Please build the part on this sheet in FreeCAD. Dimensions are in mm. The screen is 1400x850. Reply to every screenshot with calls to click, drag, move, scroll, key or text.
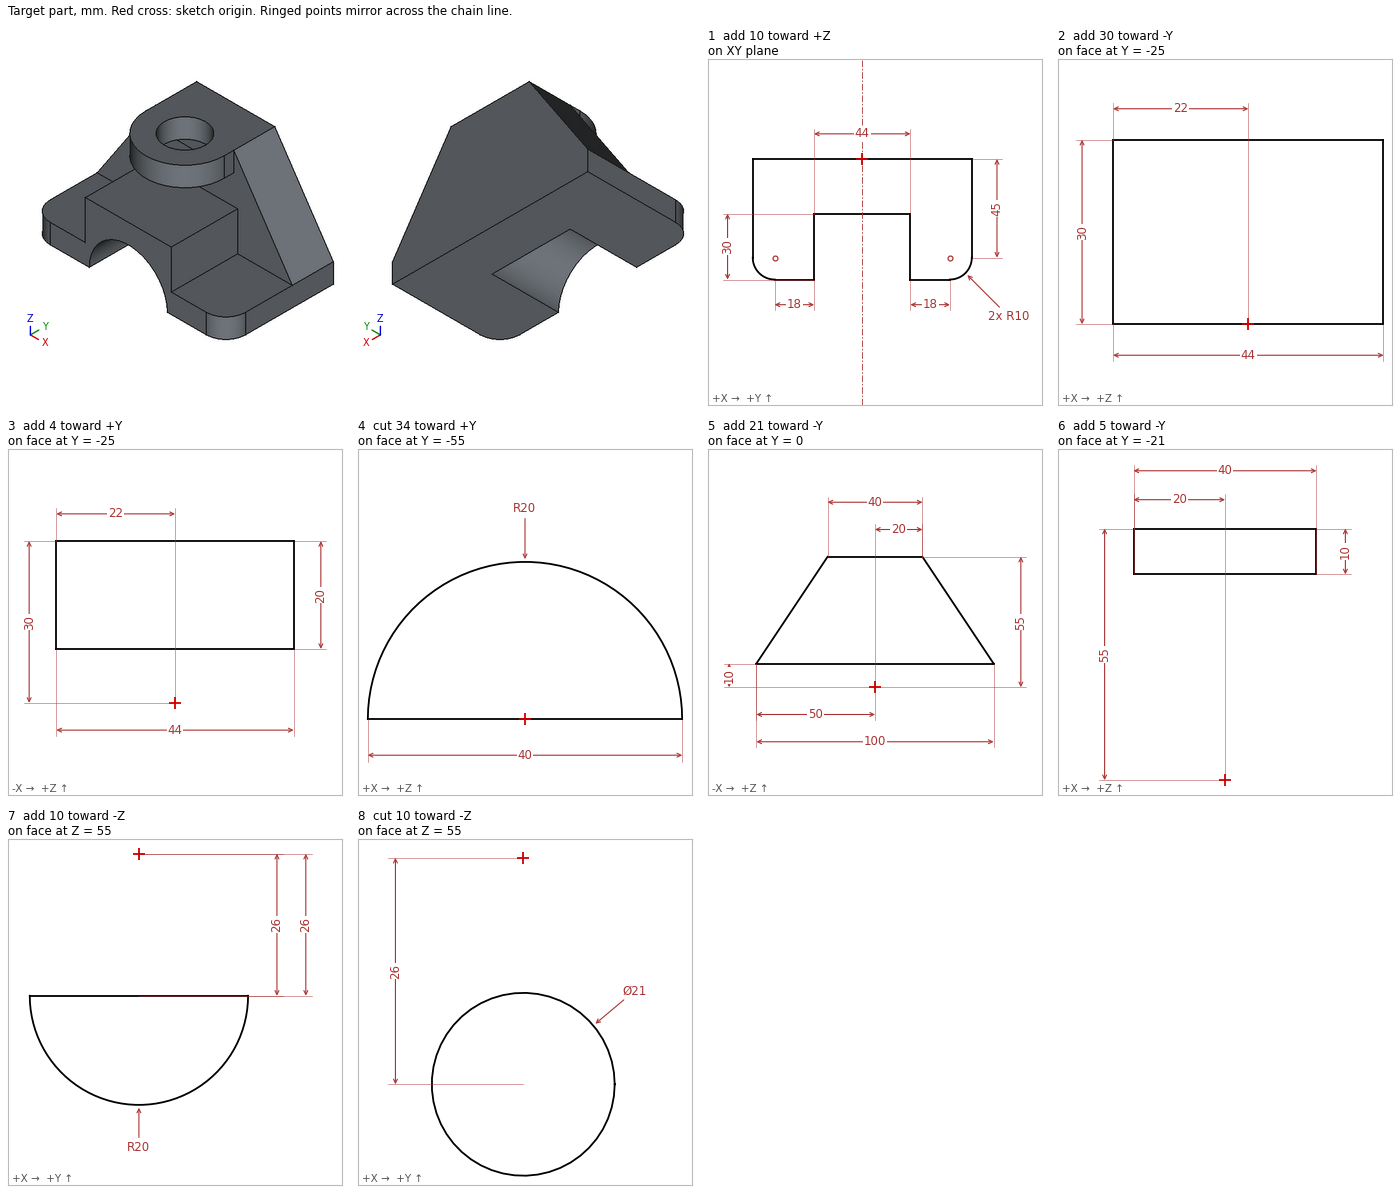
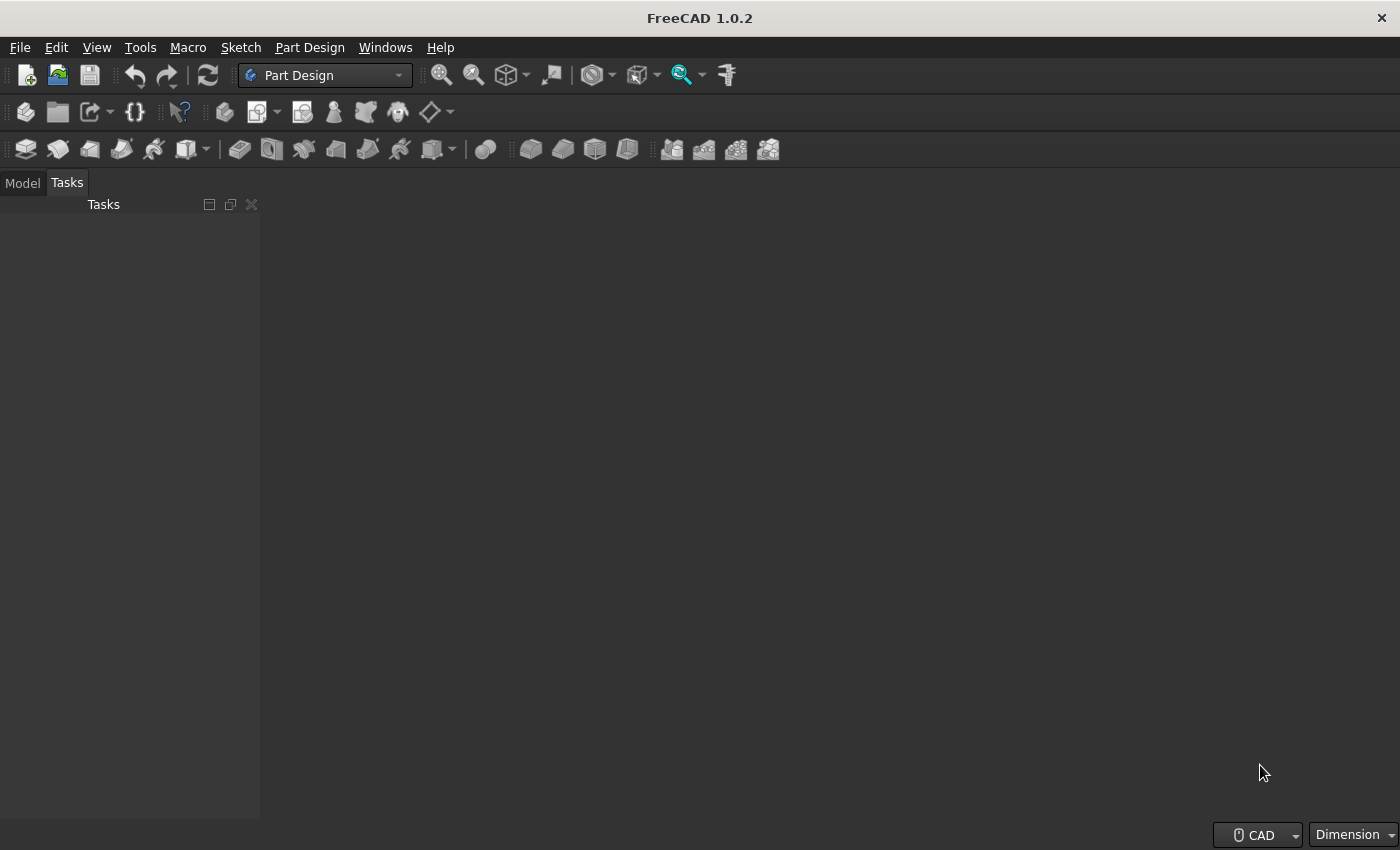
click(26, 76)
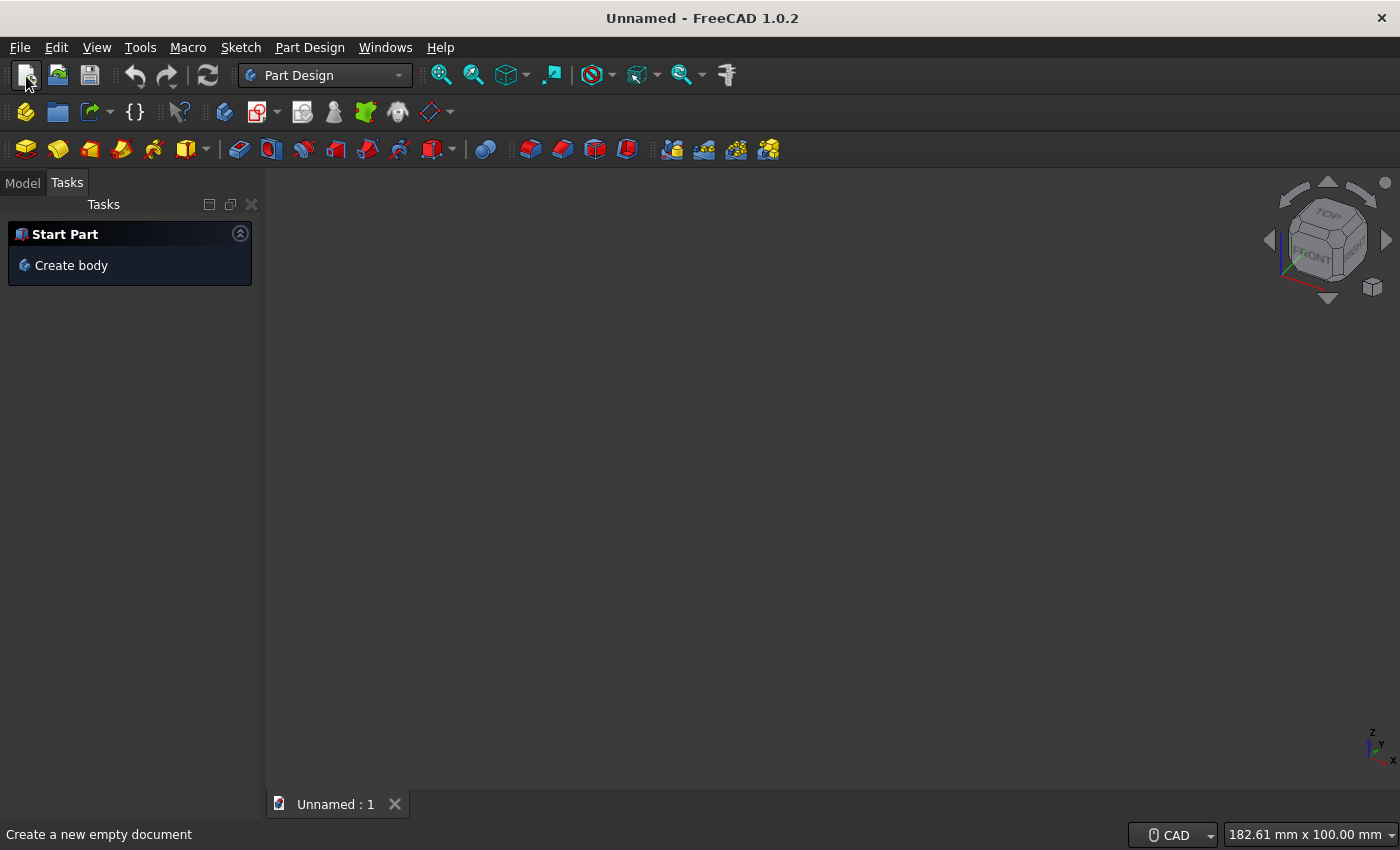
click(258, 112)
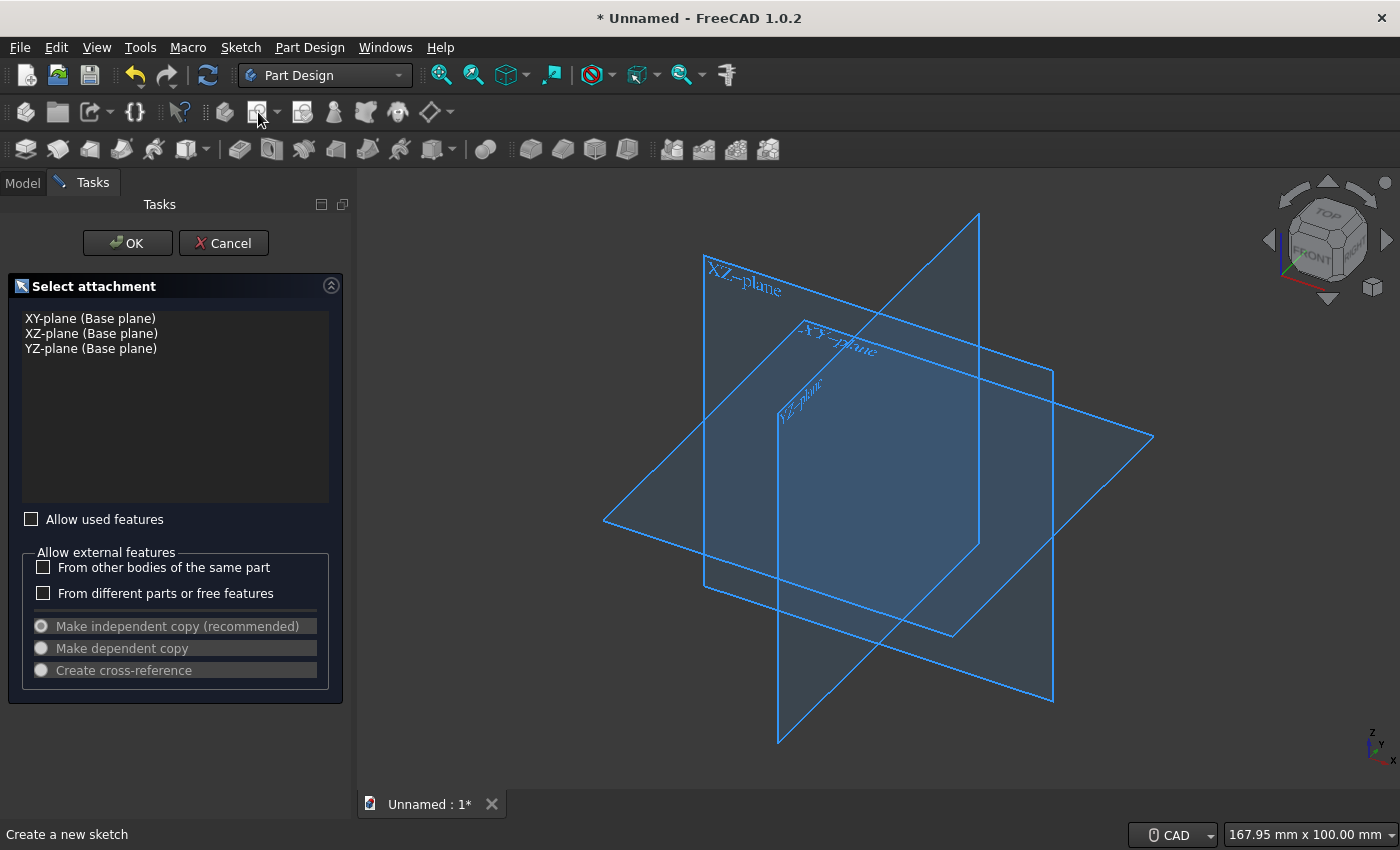
click(82, 318)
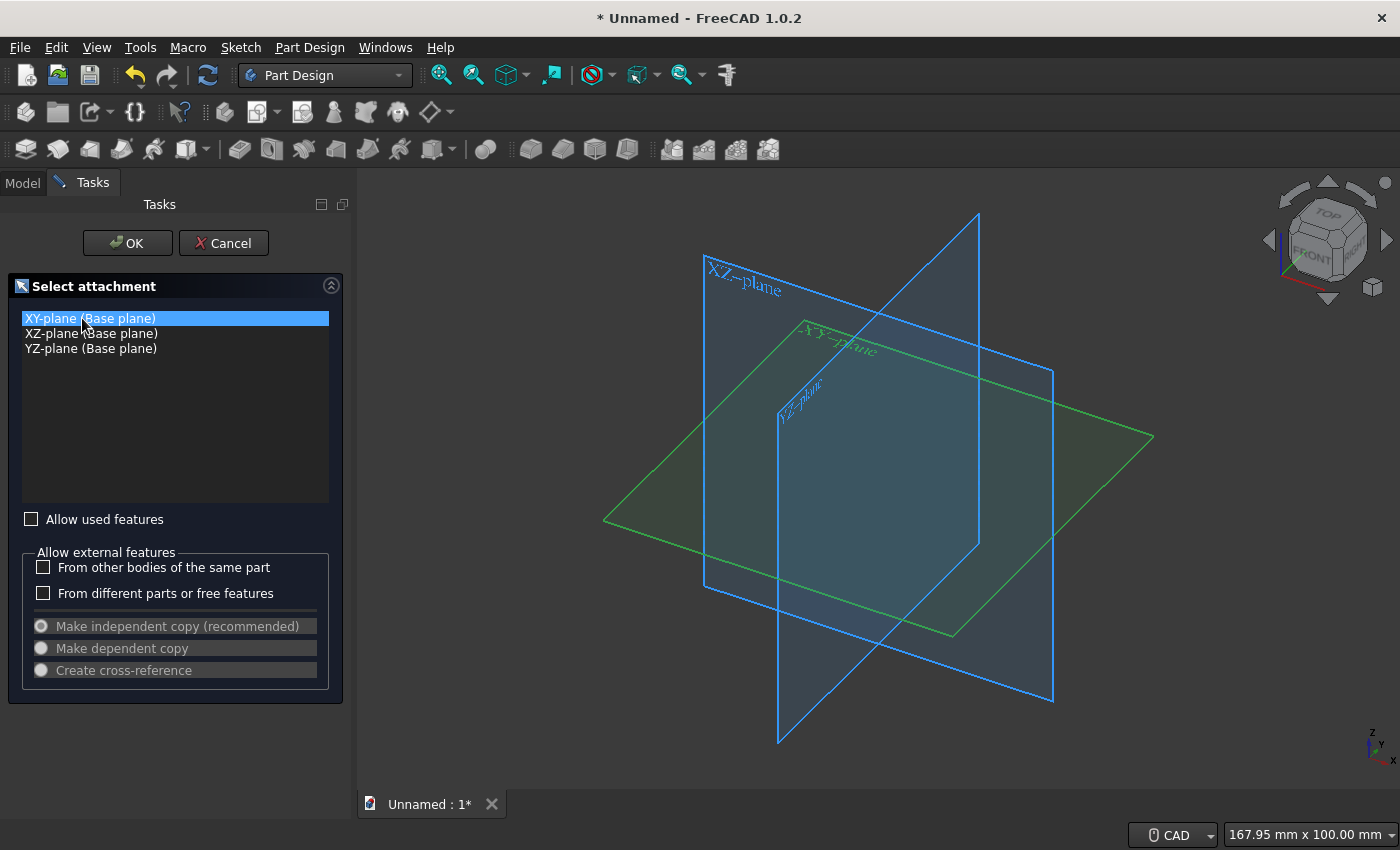
click(128, 243)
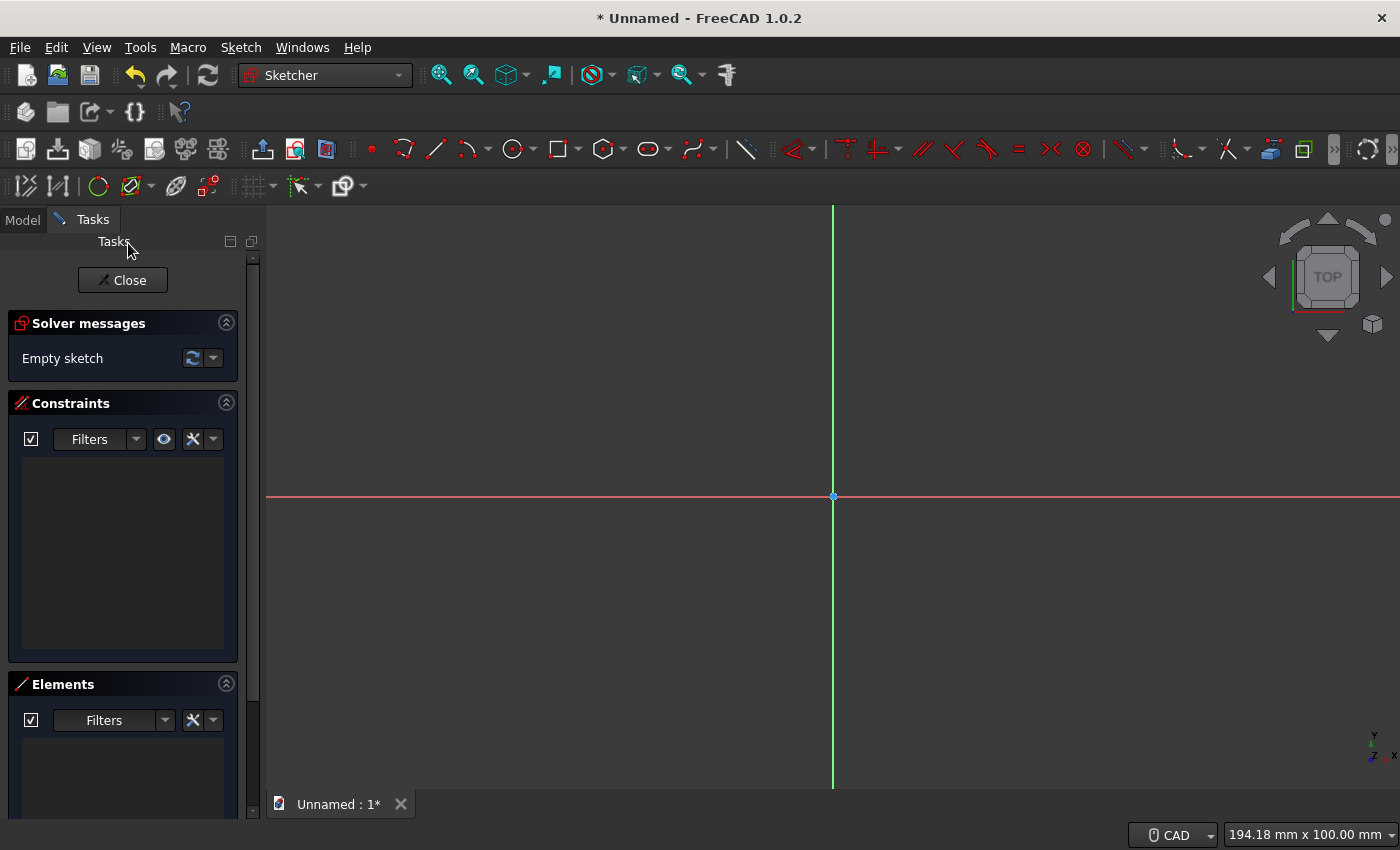
scroll(455, 233, down, 1)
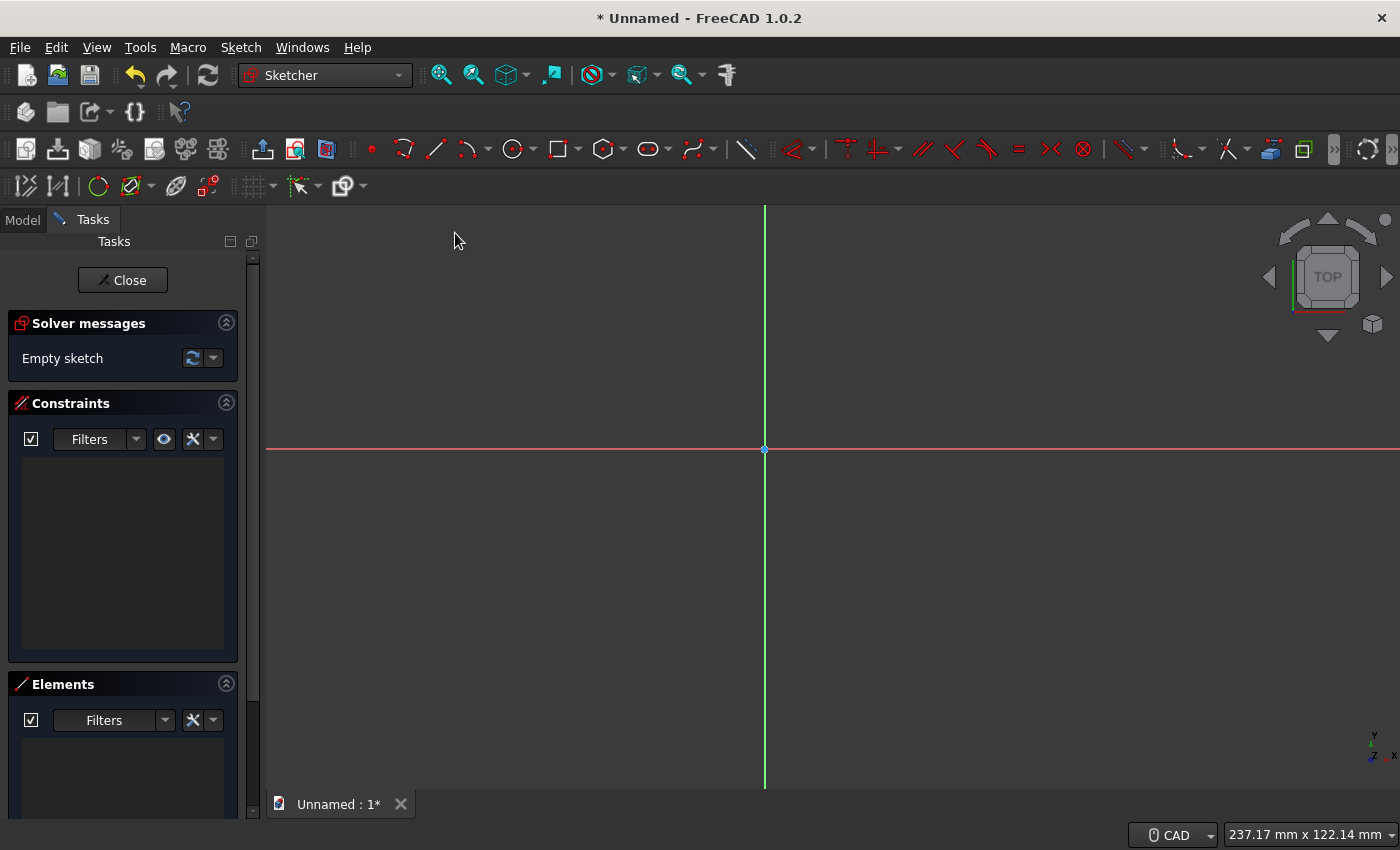
scroll(765, 751, up, 2)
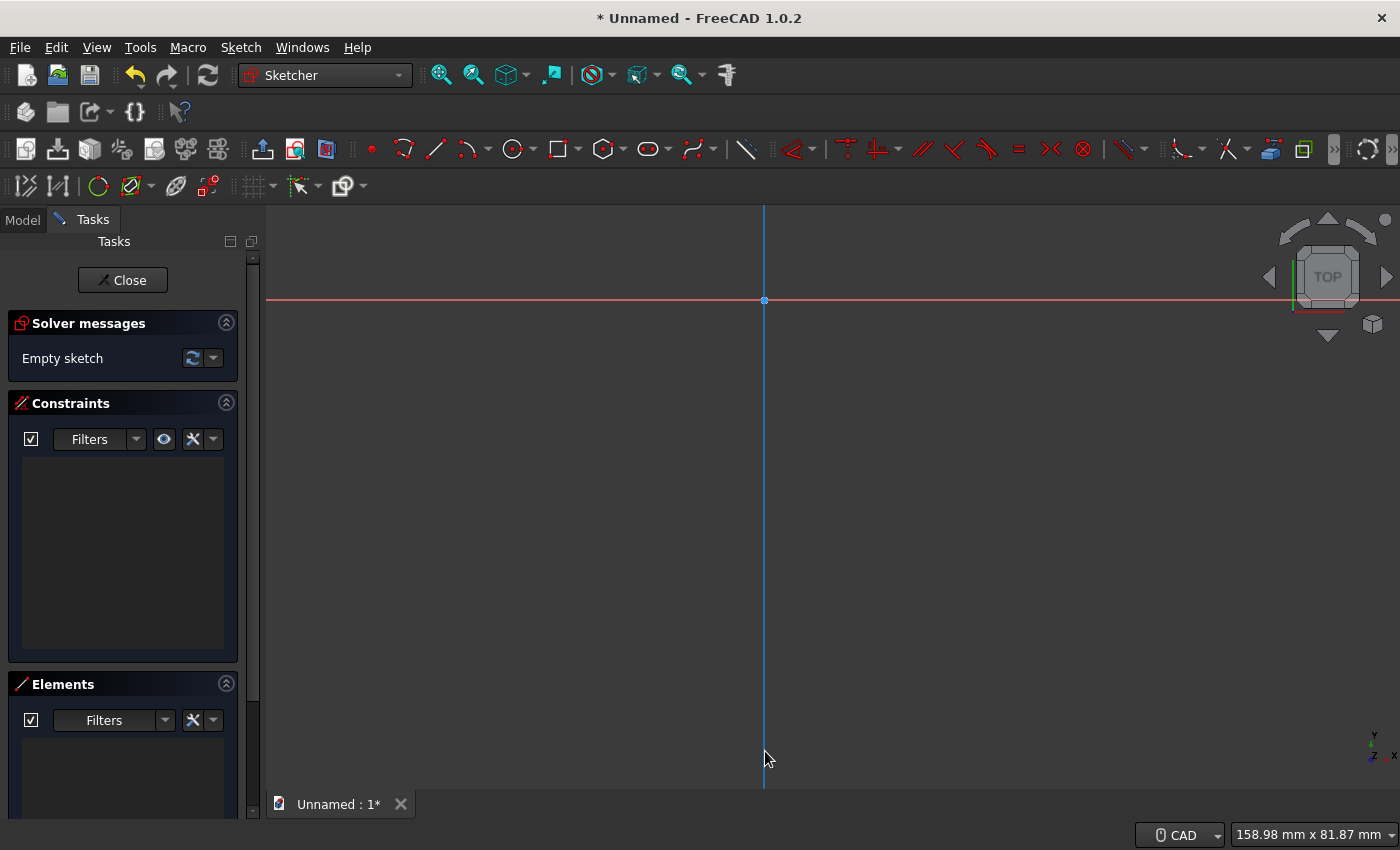
click(404, 150)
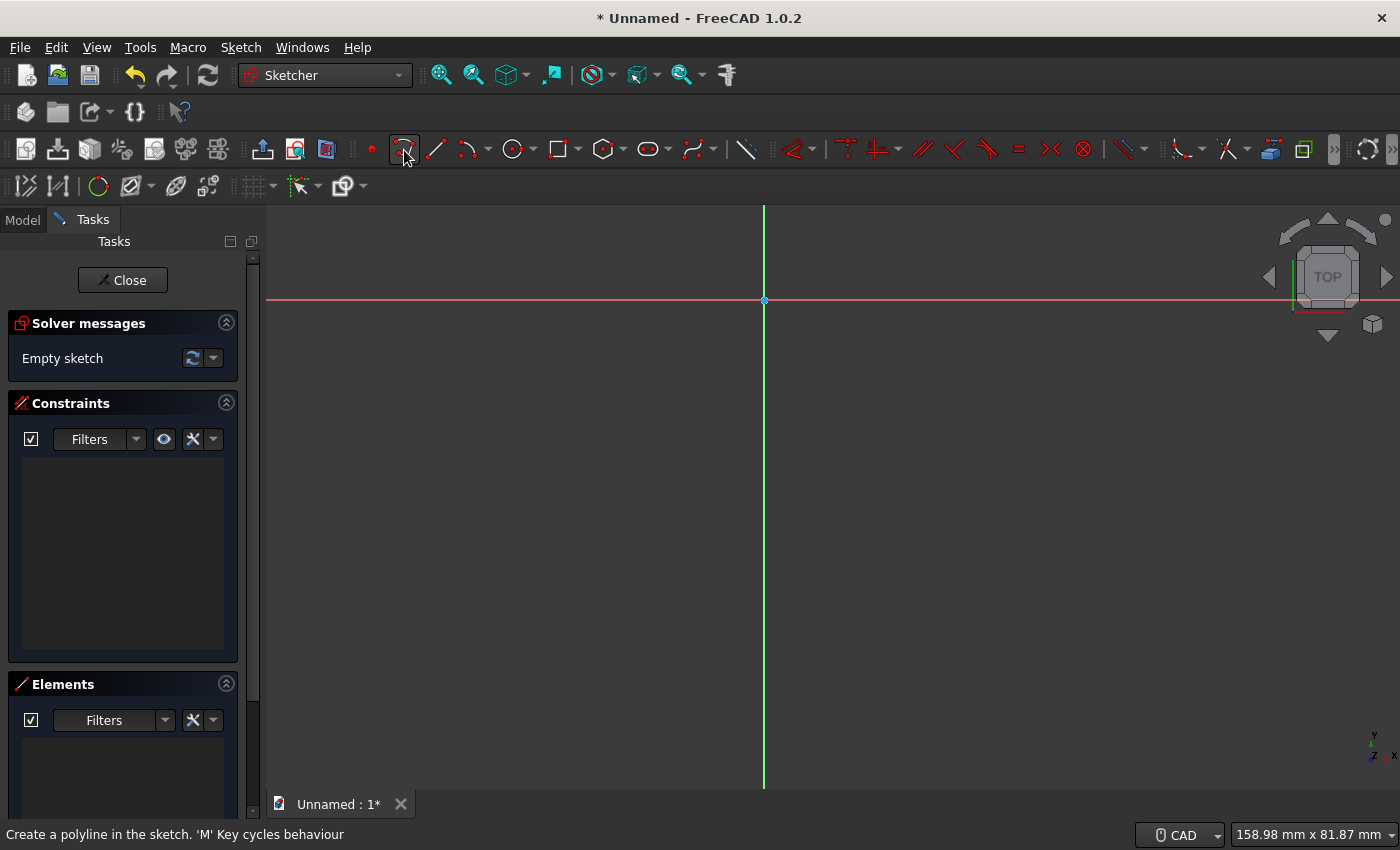
click(1121, 621)
click(1121, 300)
click(407, 309)
click(407, 621)
right_click(407, 621)